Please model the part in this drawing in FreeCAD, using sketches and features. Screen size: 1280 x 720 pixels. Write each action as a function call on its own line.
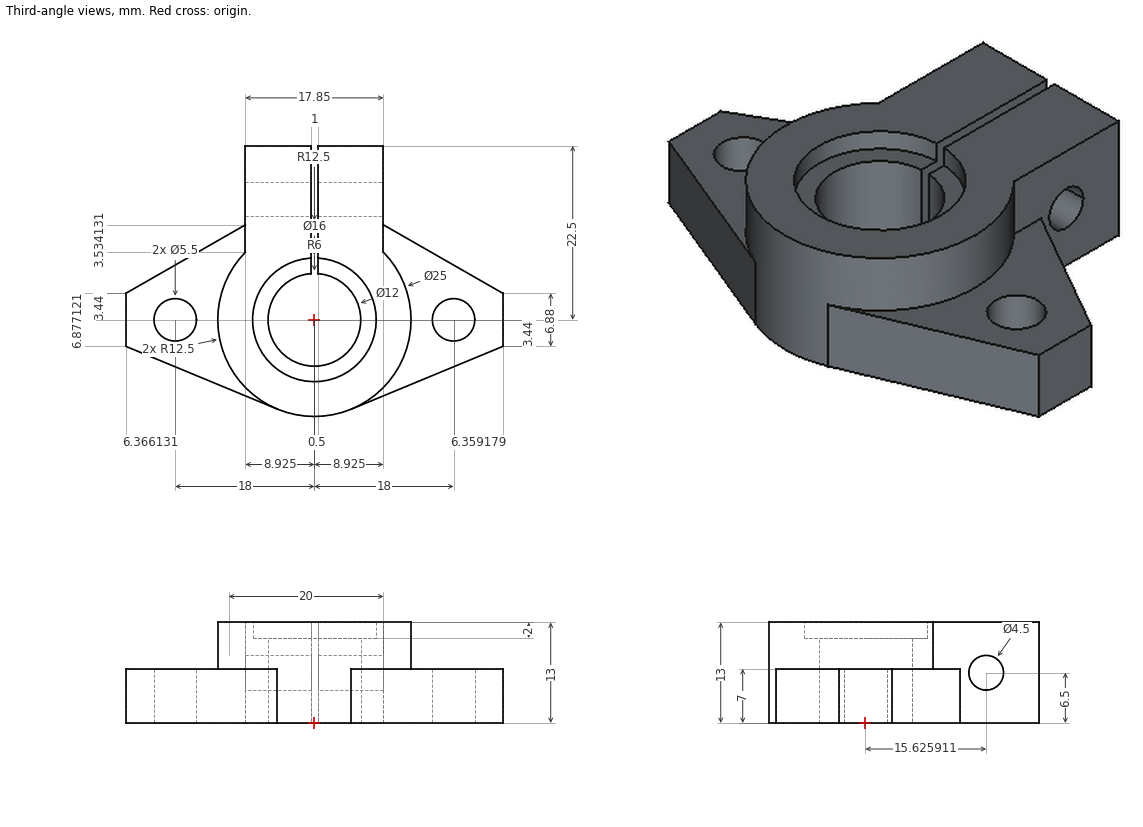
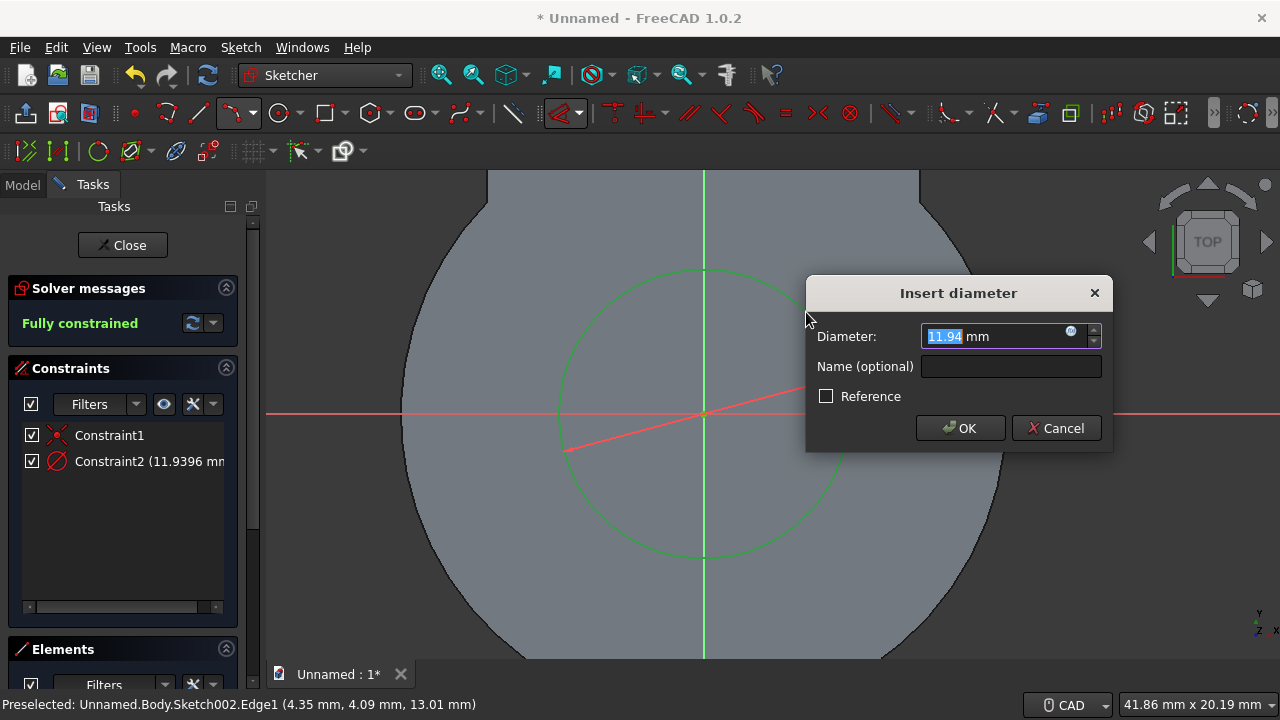
text(12)
key(Return)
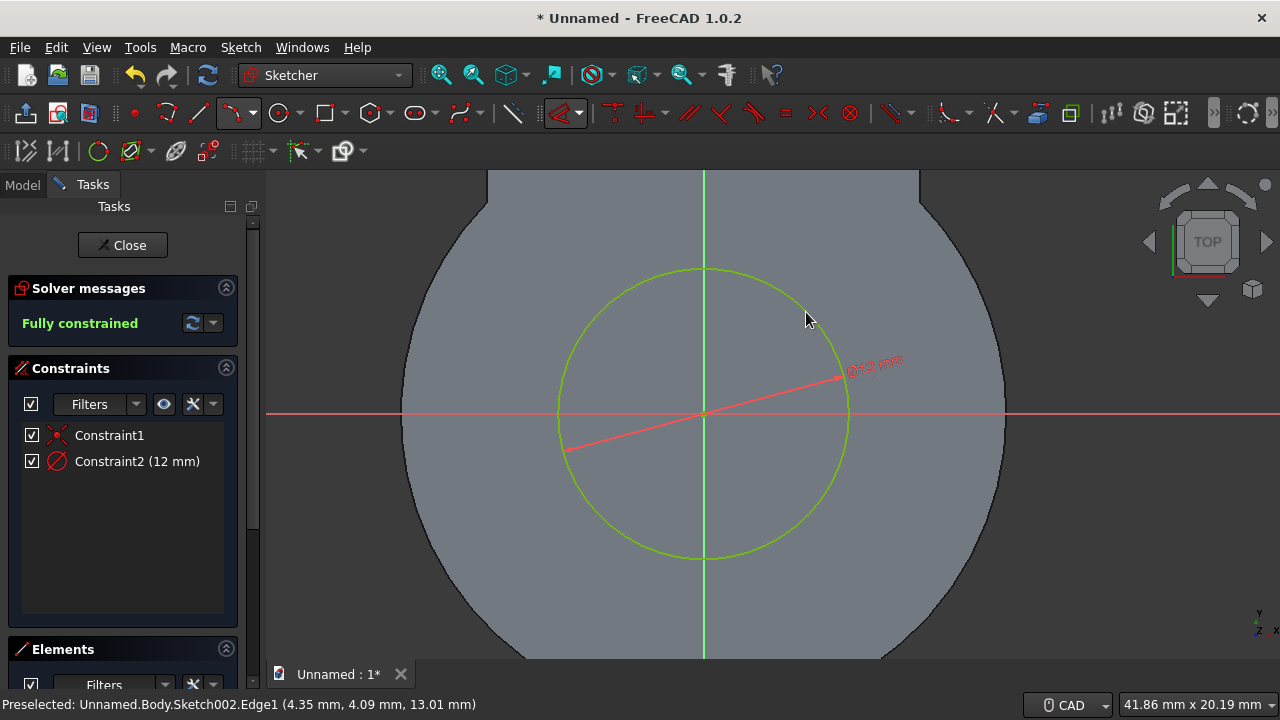
click(123, 245)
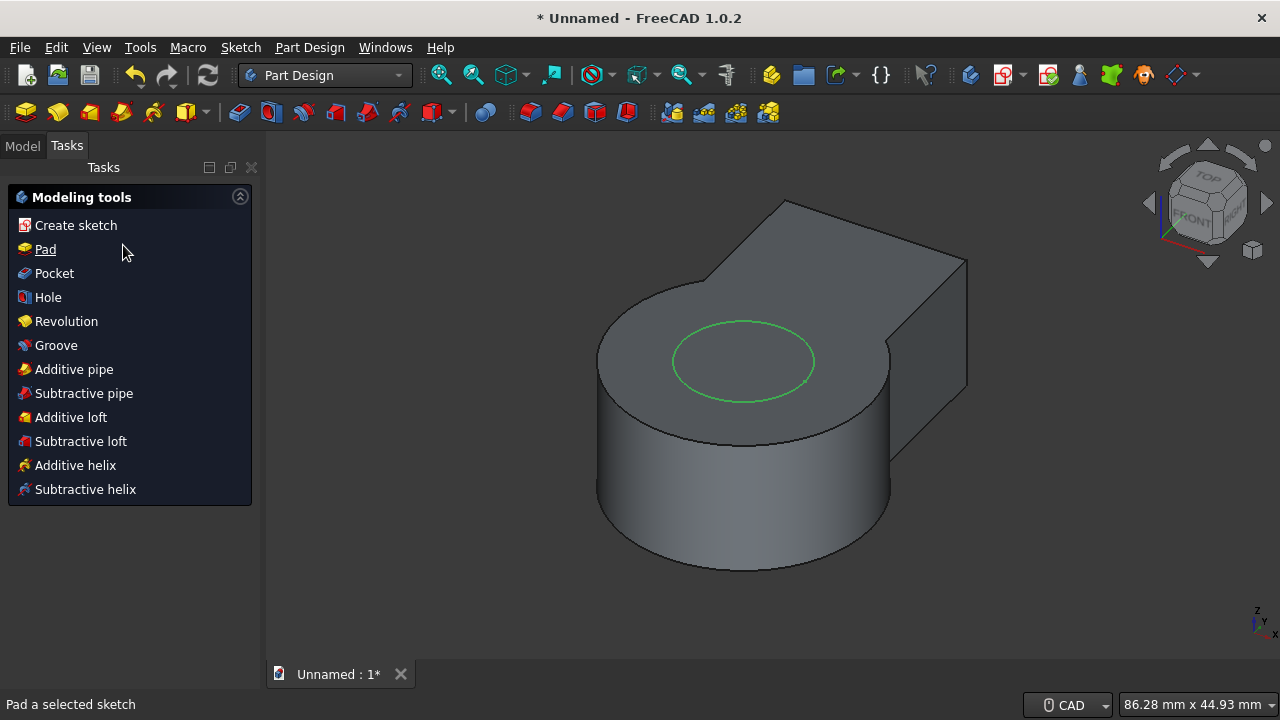
click(240, 112)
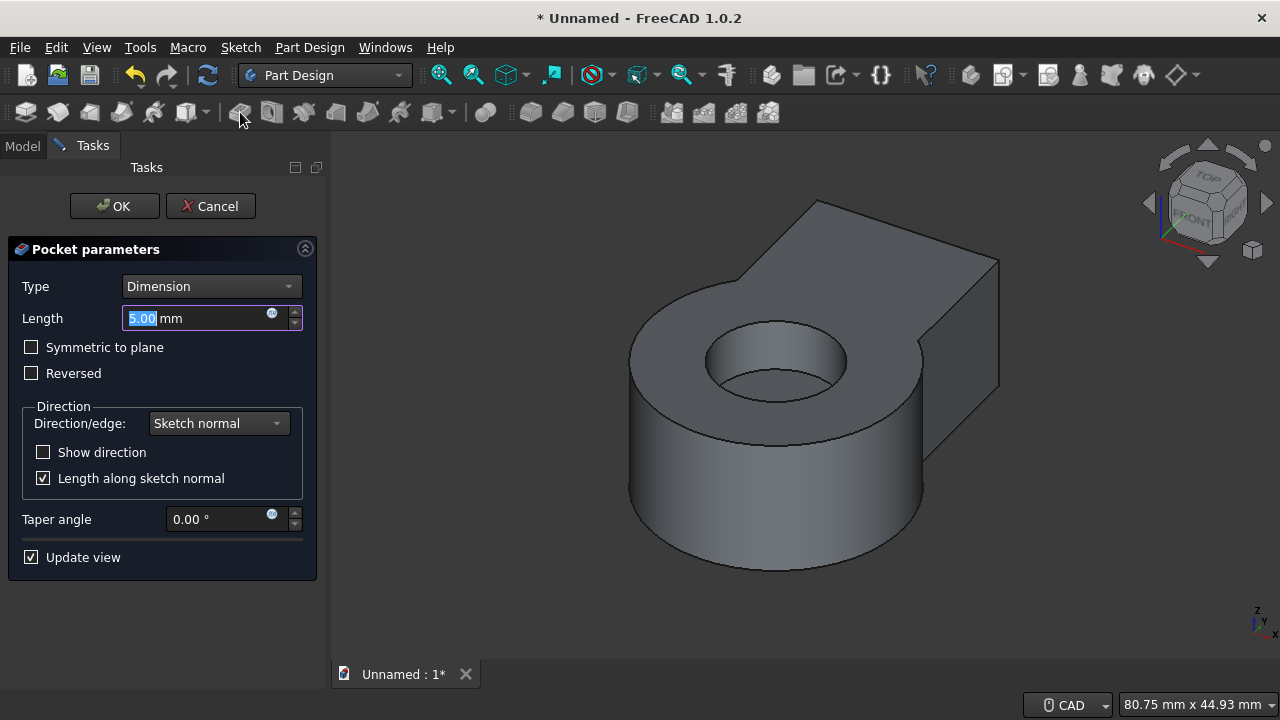
text(13)
key(Tab)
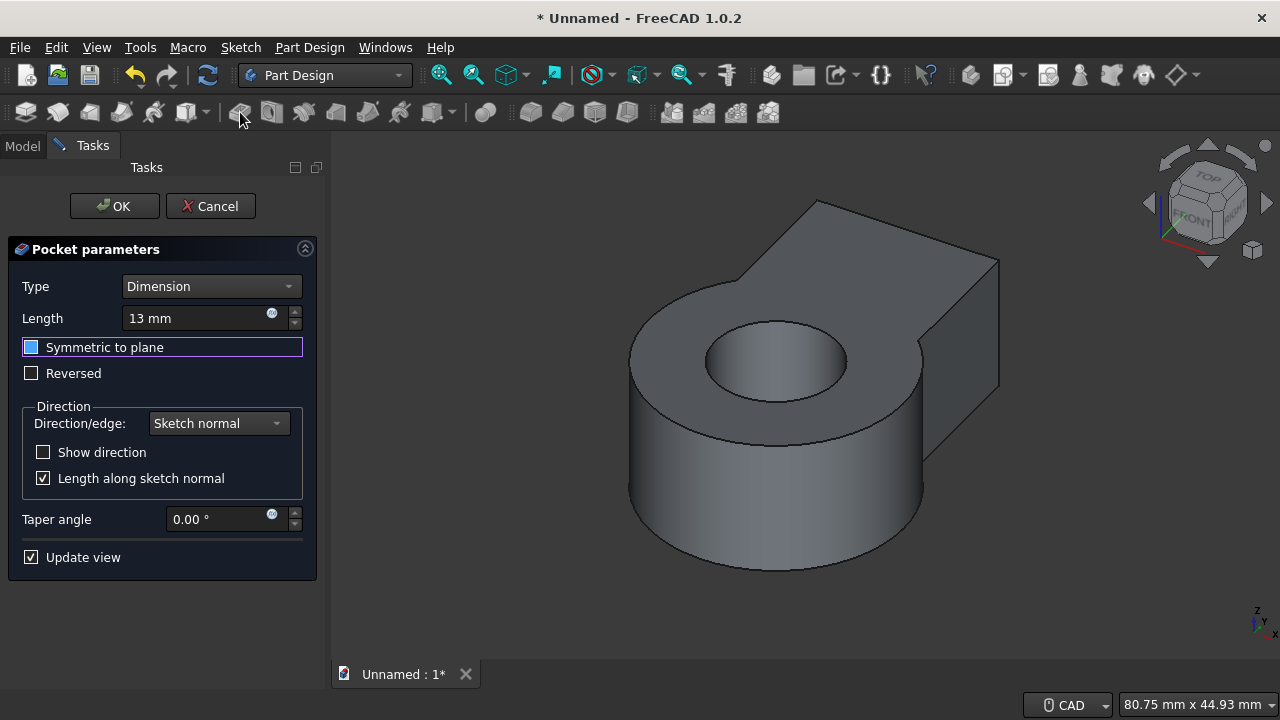
click(115, 206)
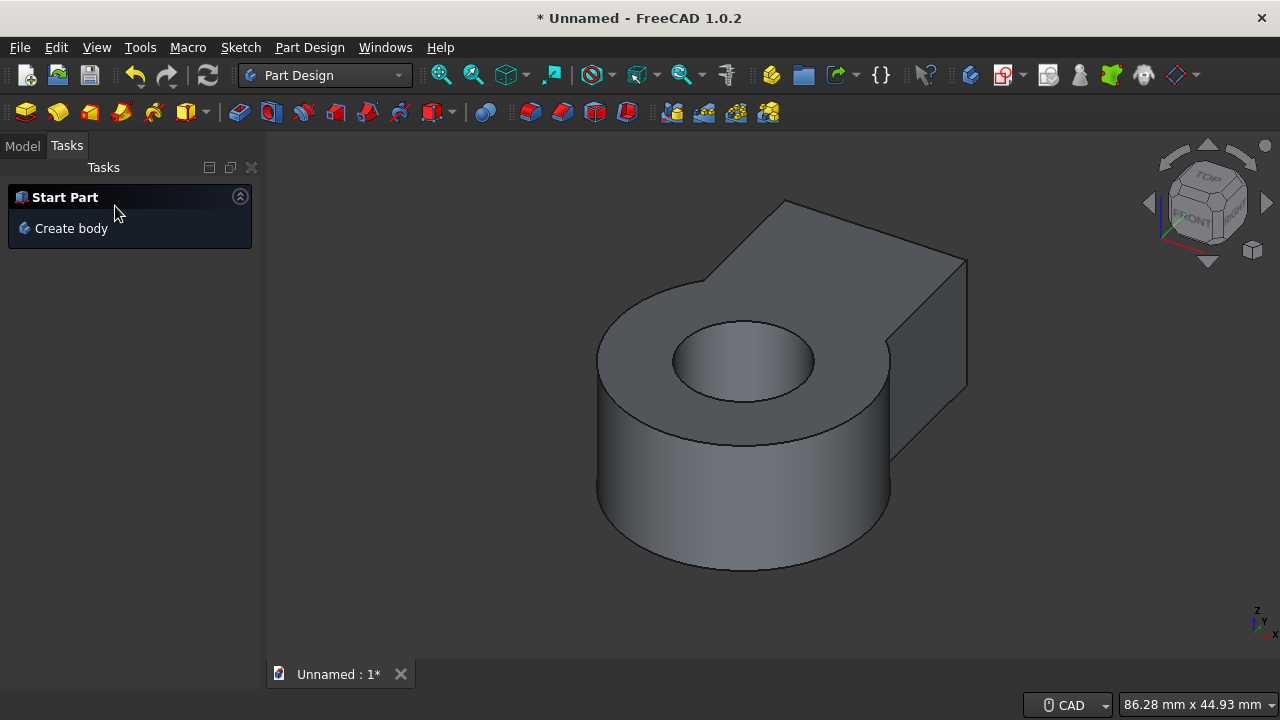
click(832, 273)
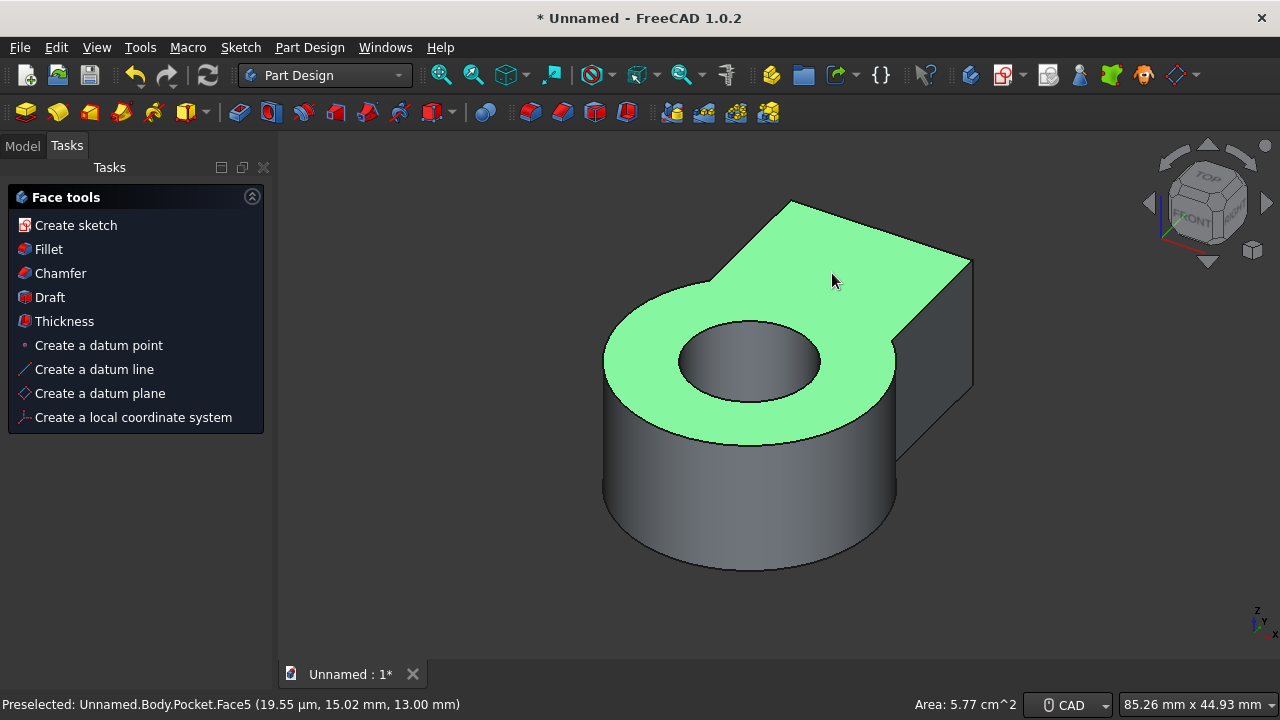
click(1004, 76)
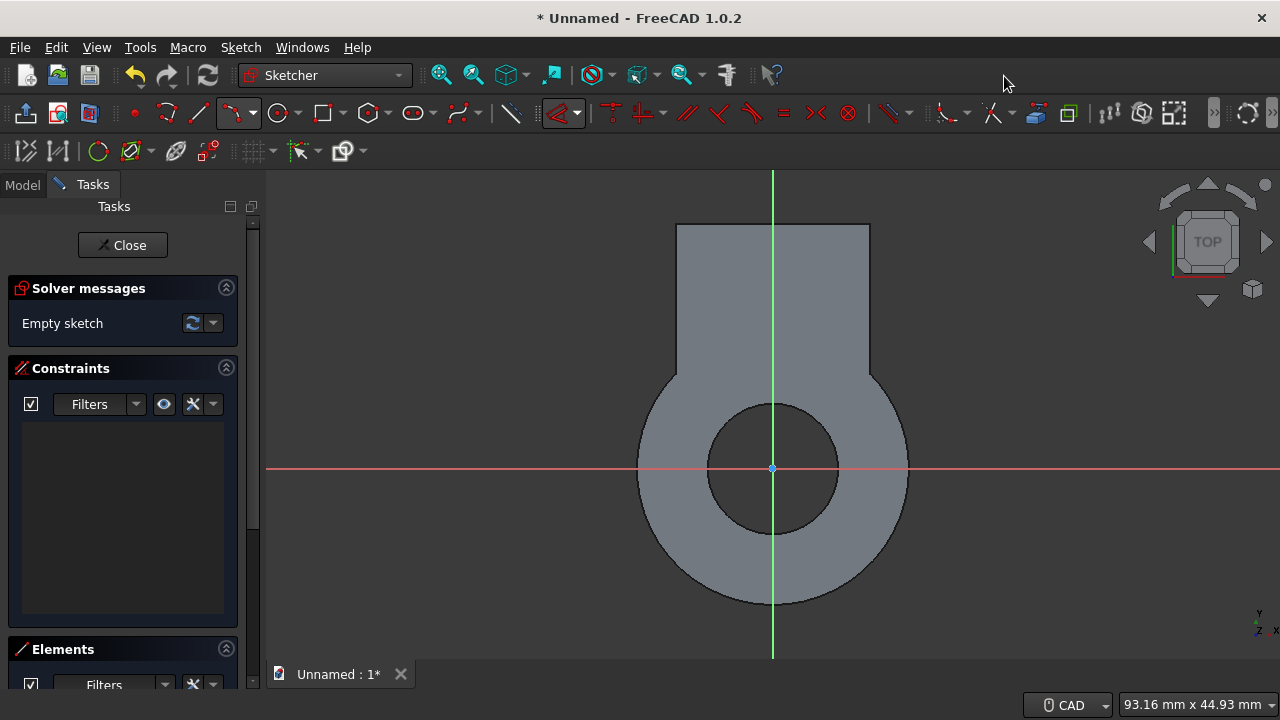
scroll(856, 535, up, 3)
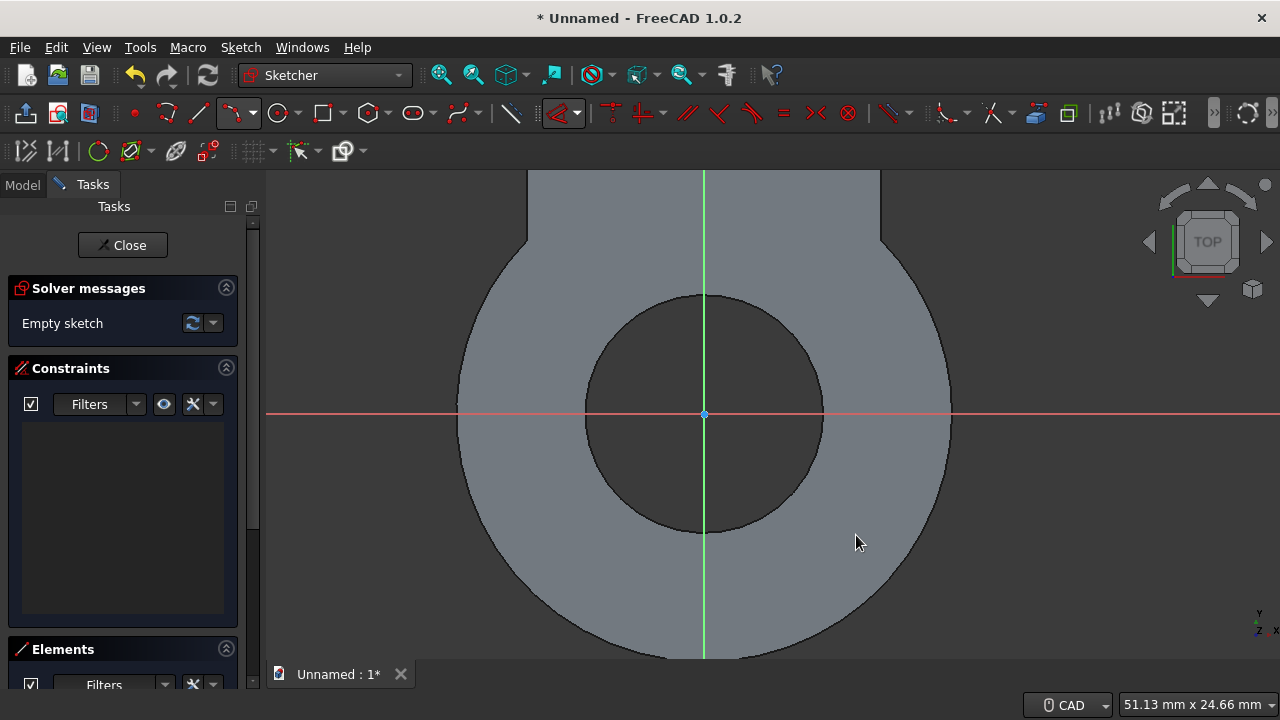
click(278, 114)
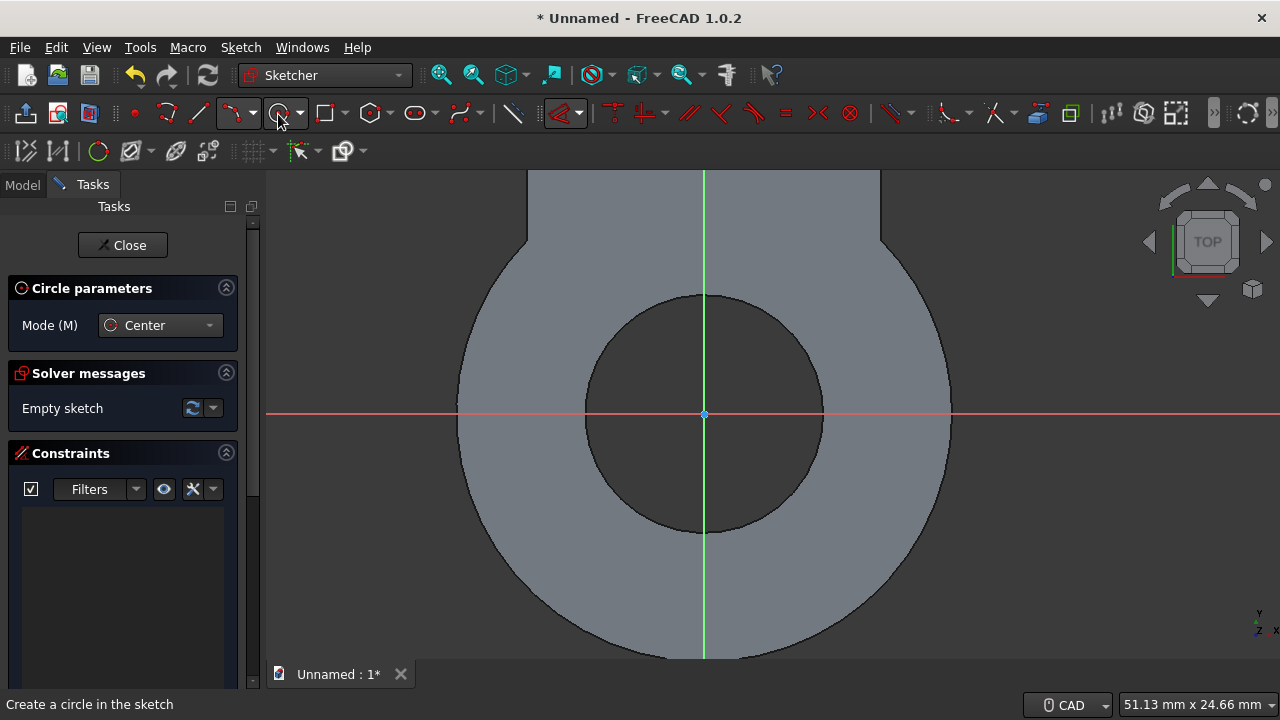
click(704, 414)
click(816, 302)
key(Escape)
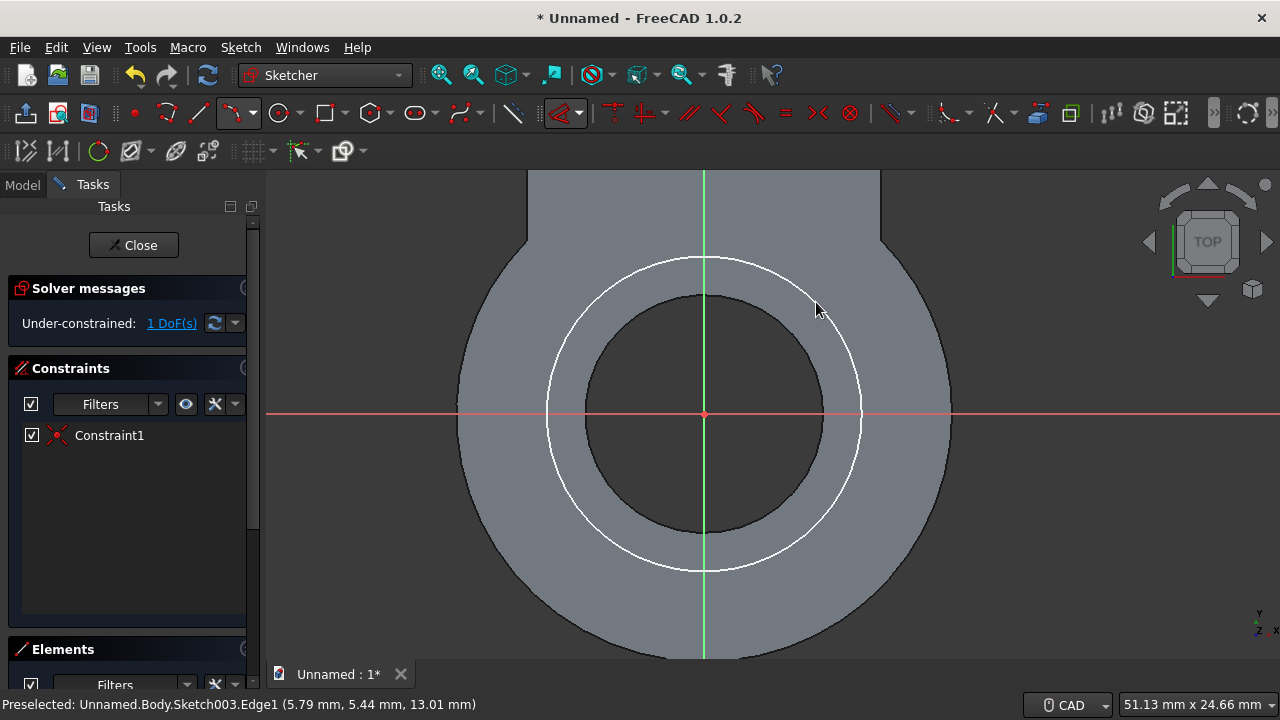
click(815, 302)